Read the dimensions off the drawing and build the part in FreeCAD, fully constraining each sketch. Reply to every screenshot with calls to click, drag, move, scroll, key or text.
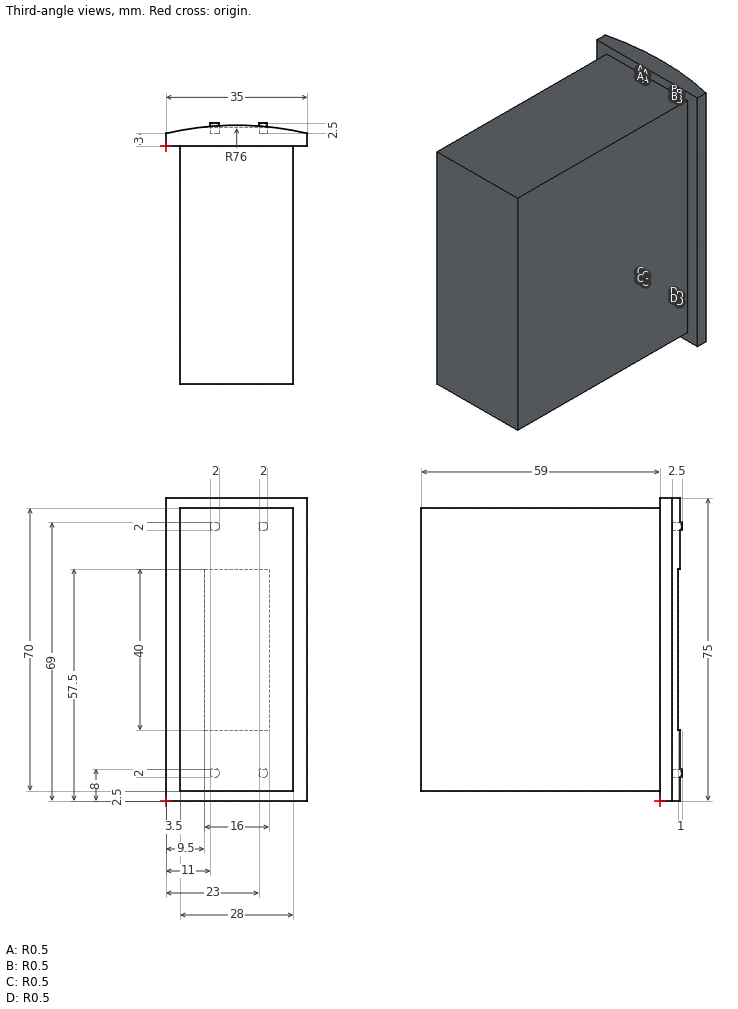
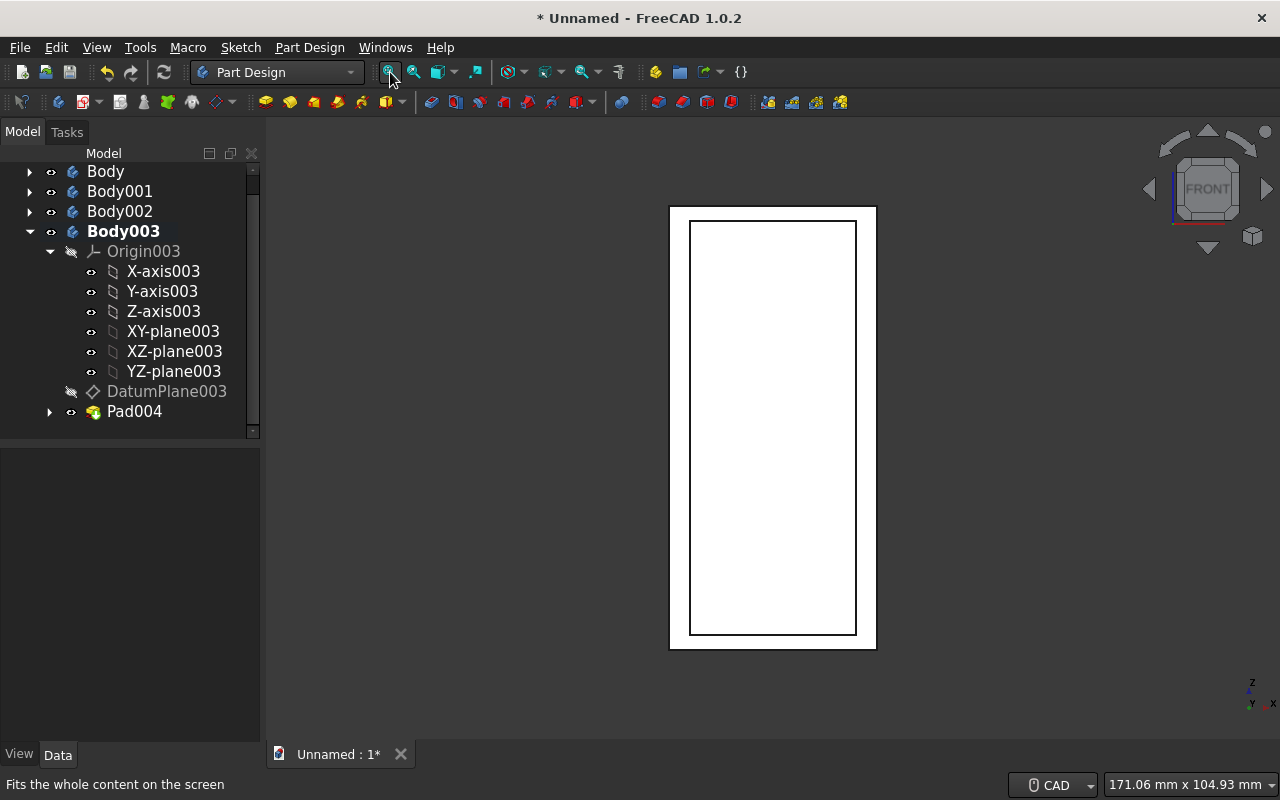
scroll(734, 602, up, 5)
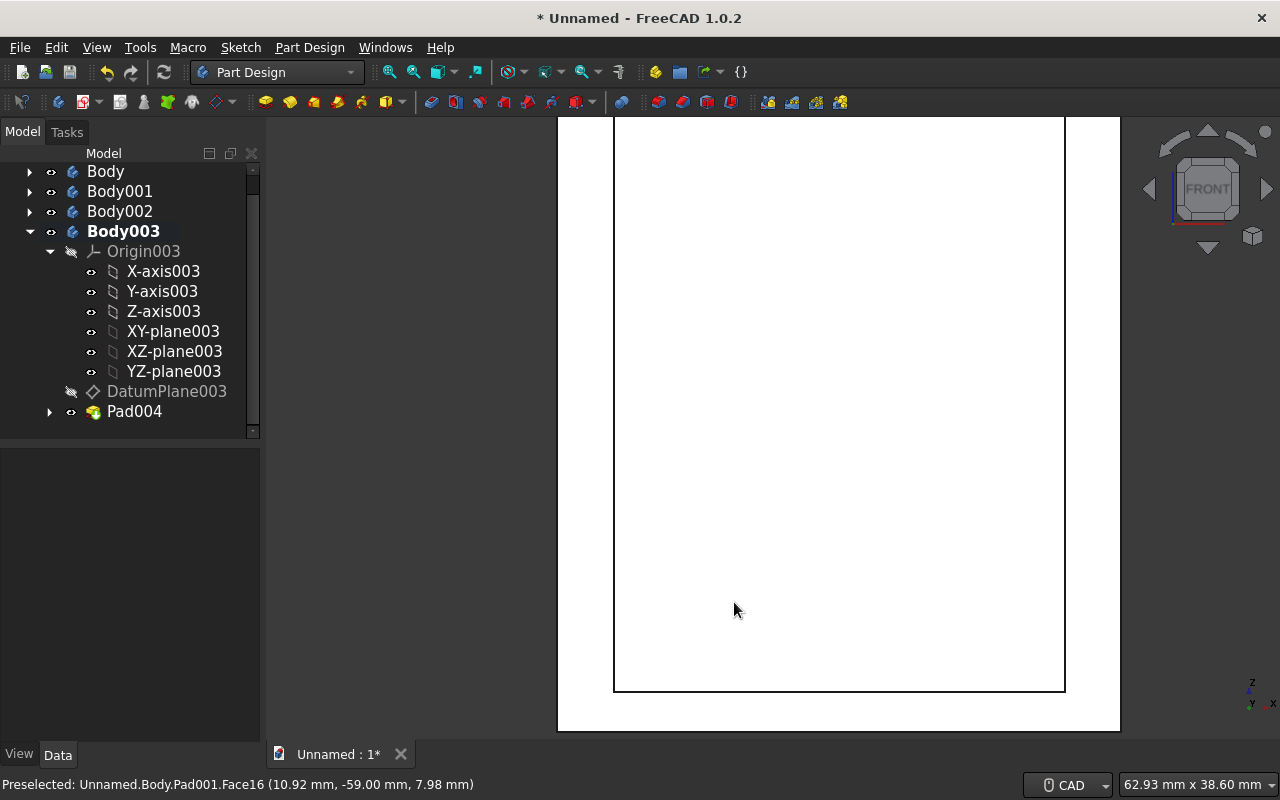
key(v)
key(f)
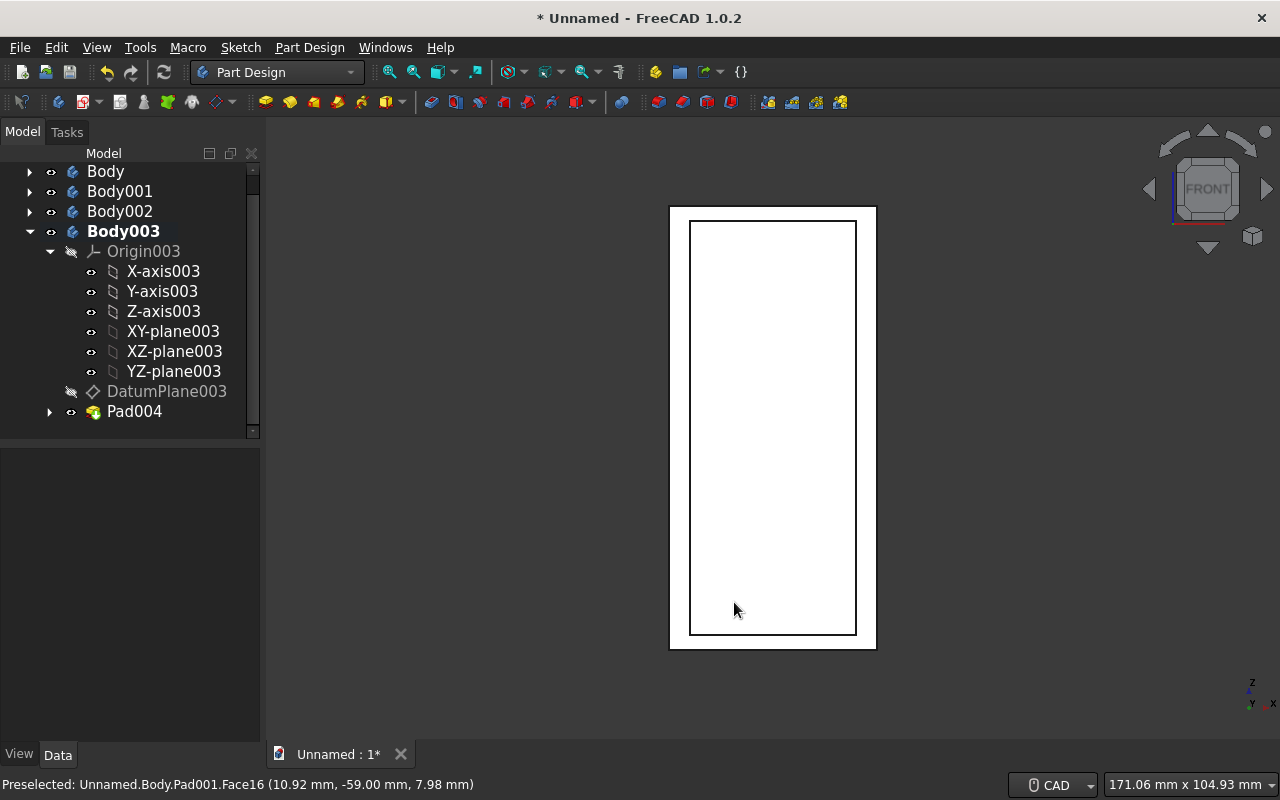
key(3)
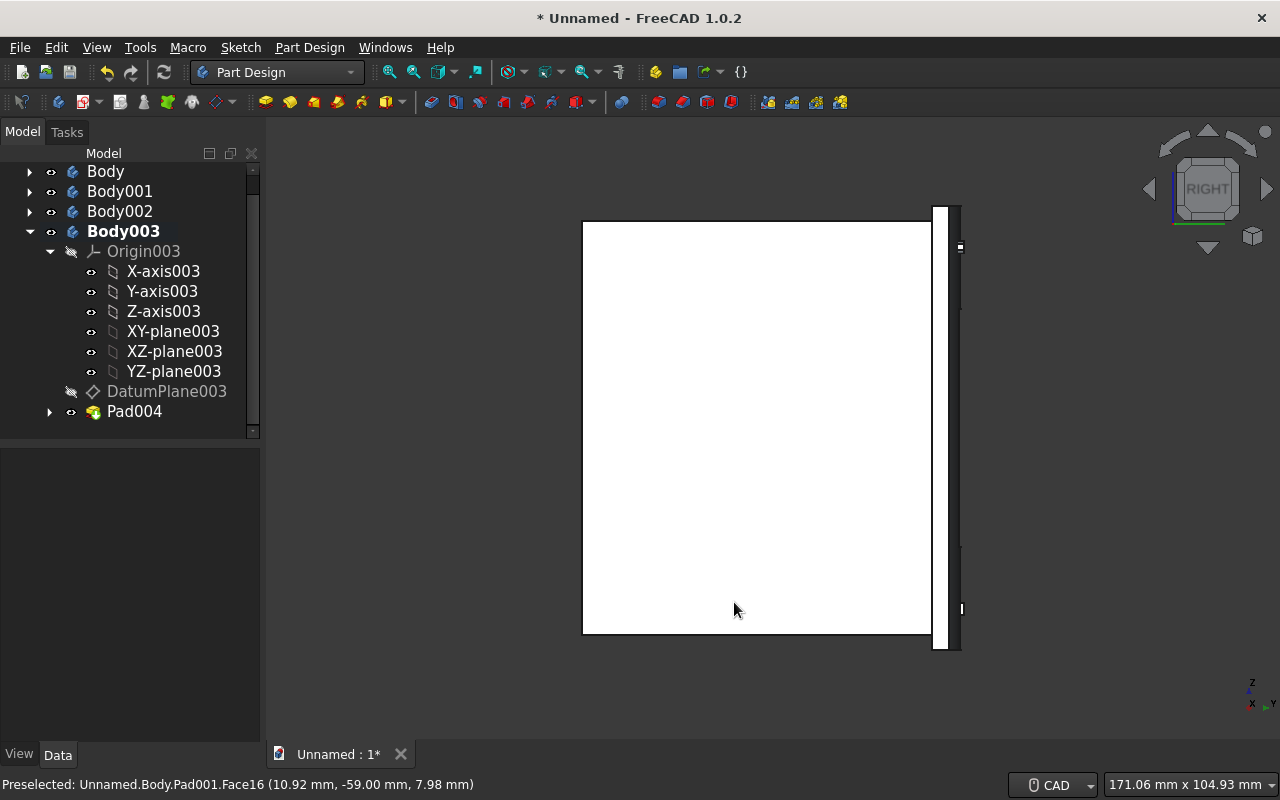
click(390, 72)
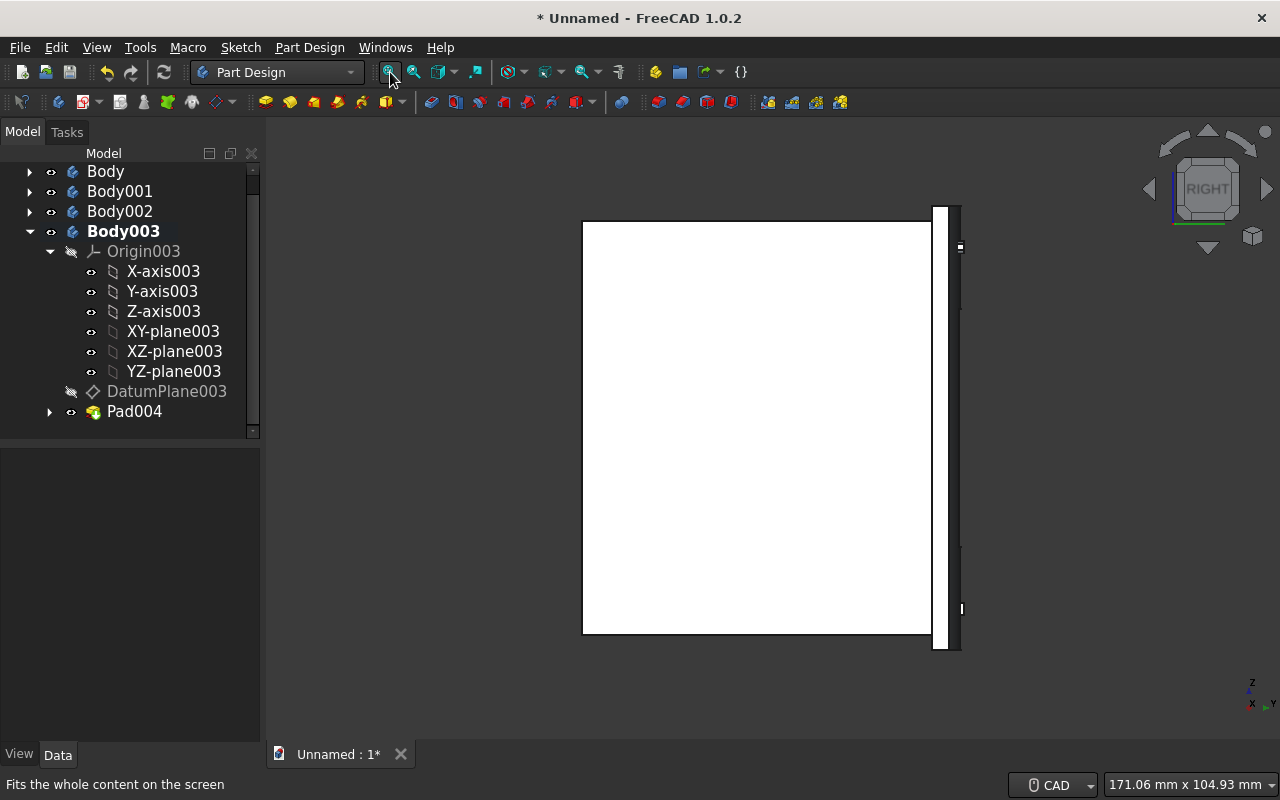
scroll(957, 602, up, 5)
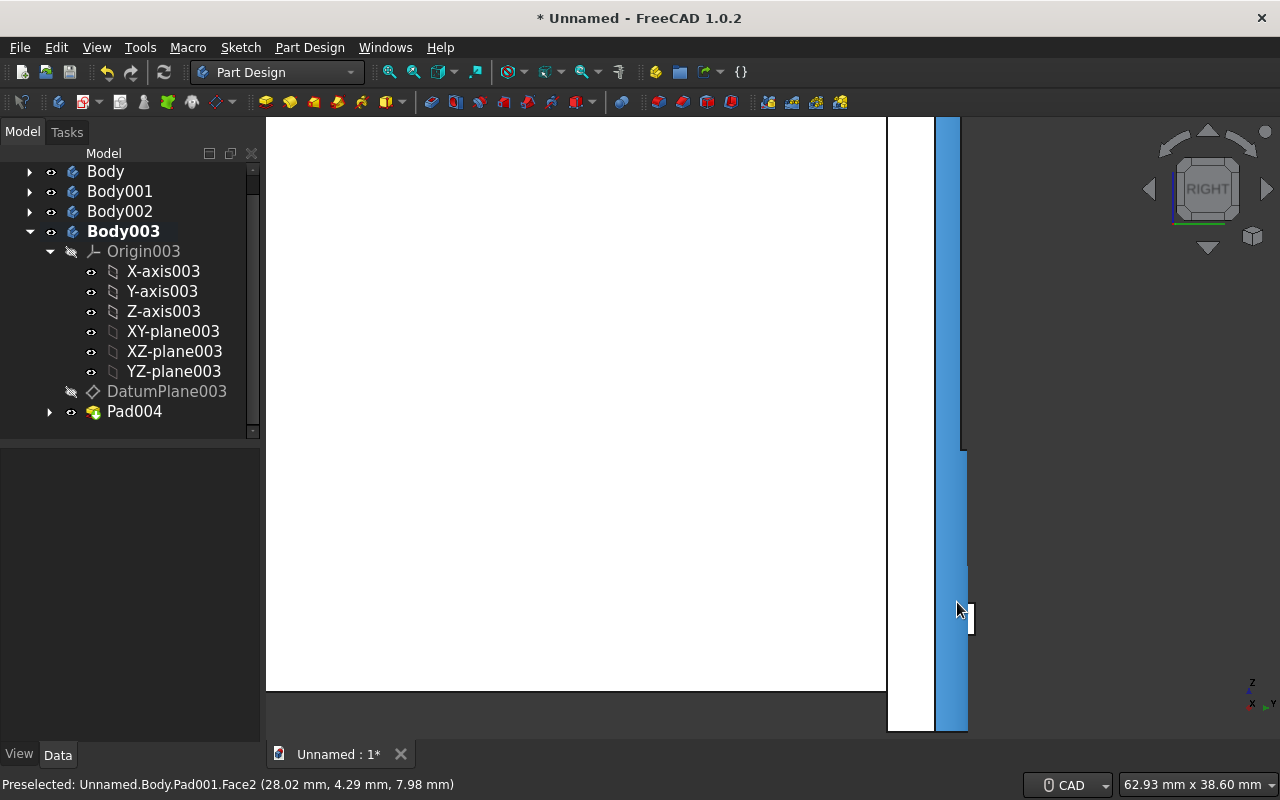
key(v)
key(f)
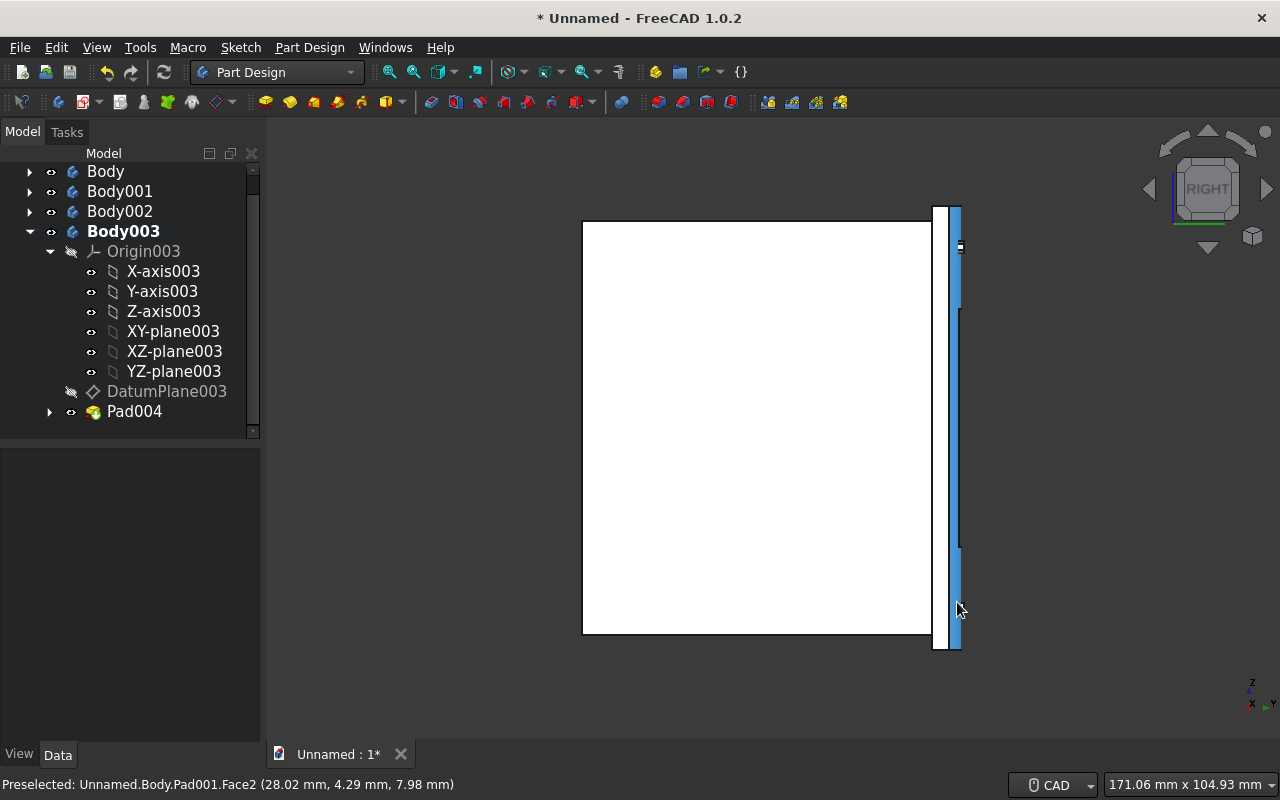
key(5)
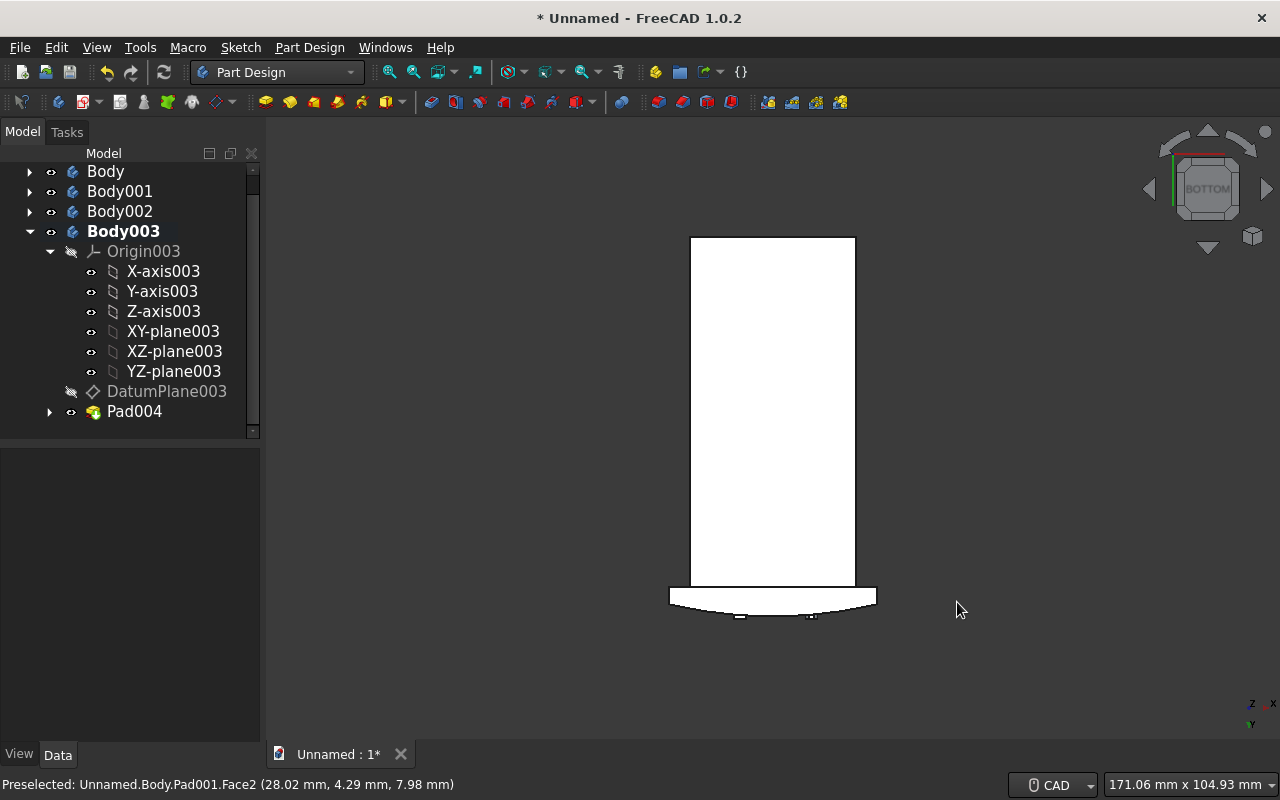
key(v)
key(f)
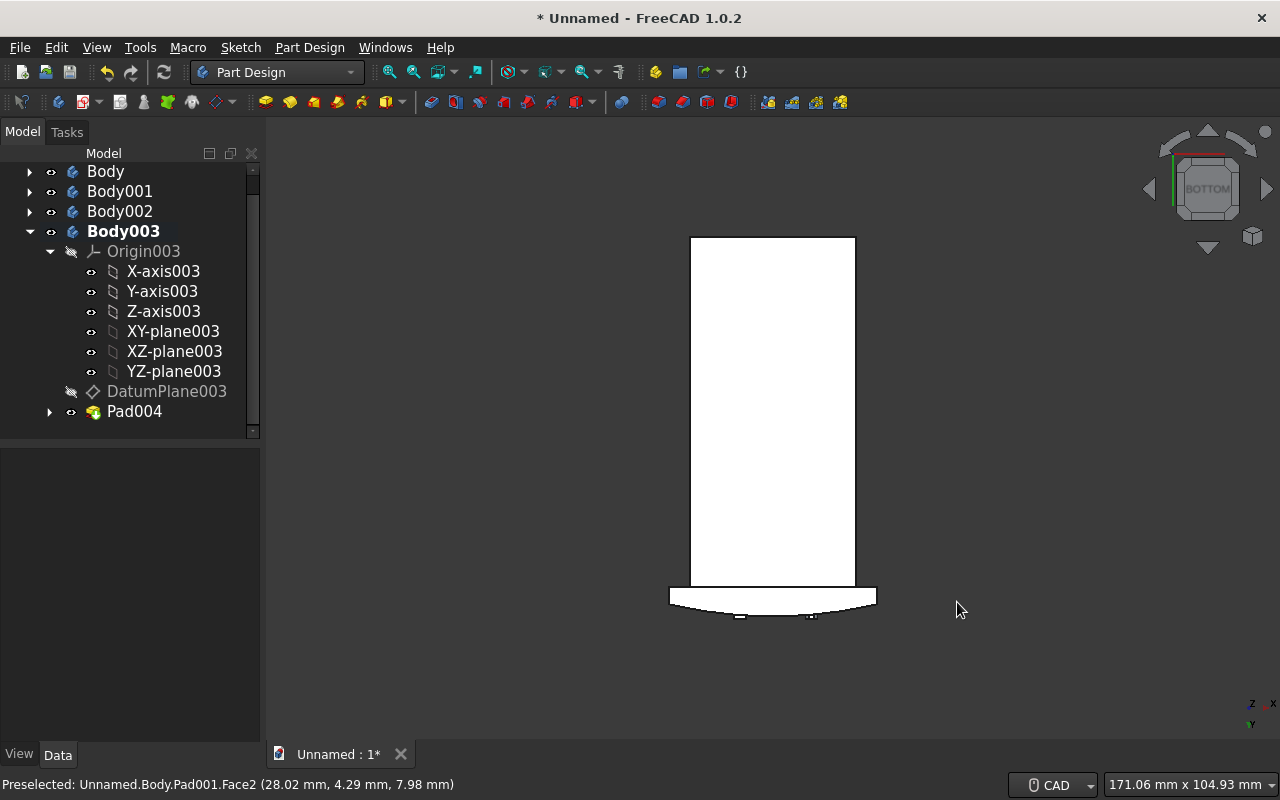
scroll(734, 611, up, 5)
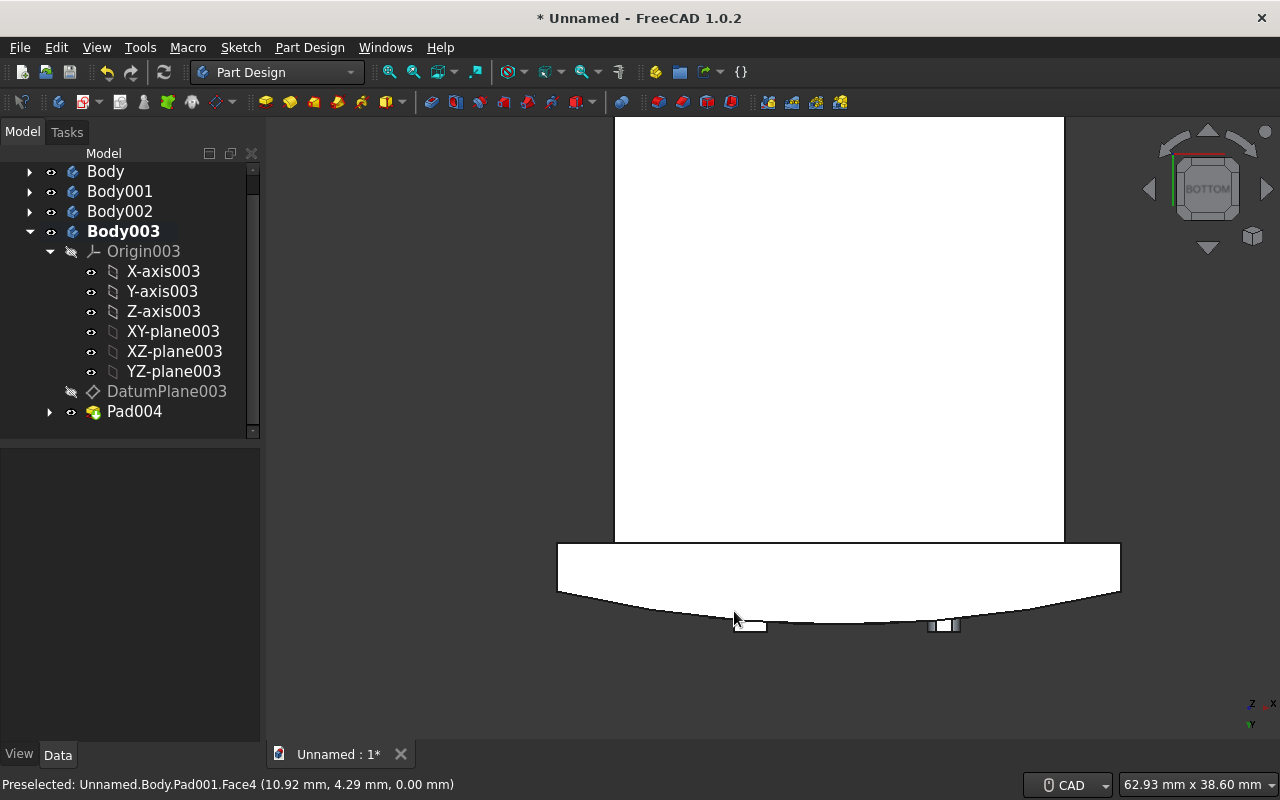
click(734, 626)